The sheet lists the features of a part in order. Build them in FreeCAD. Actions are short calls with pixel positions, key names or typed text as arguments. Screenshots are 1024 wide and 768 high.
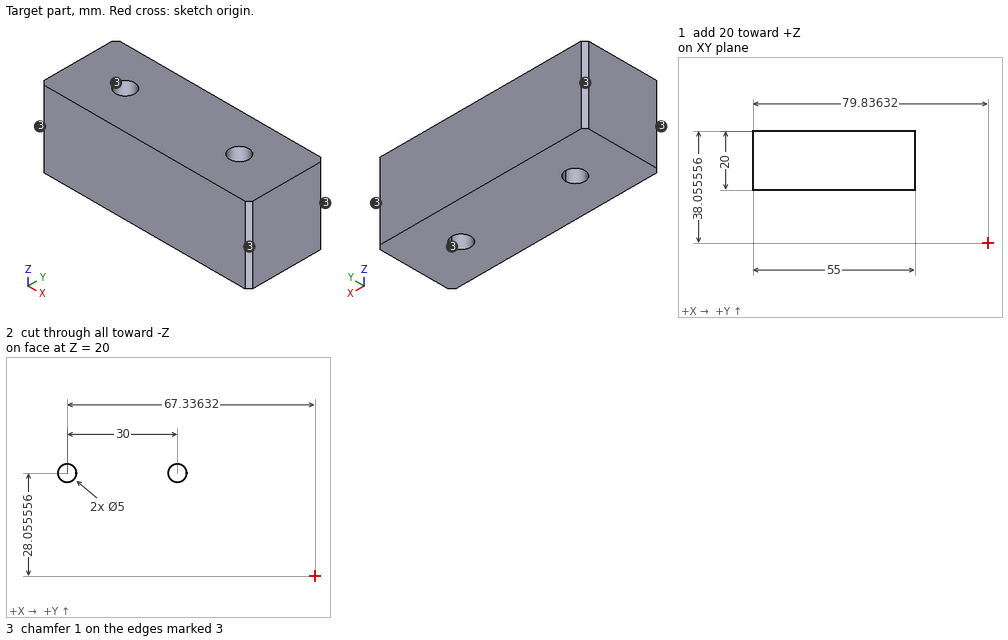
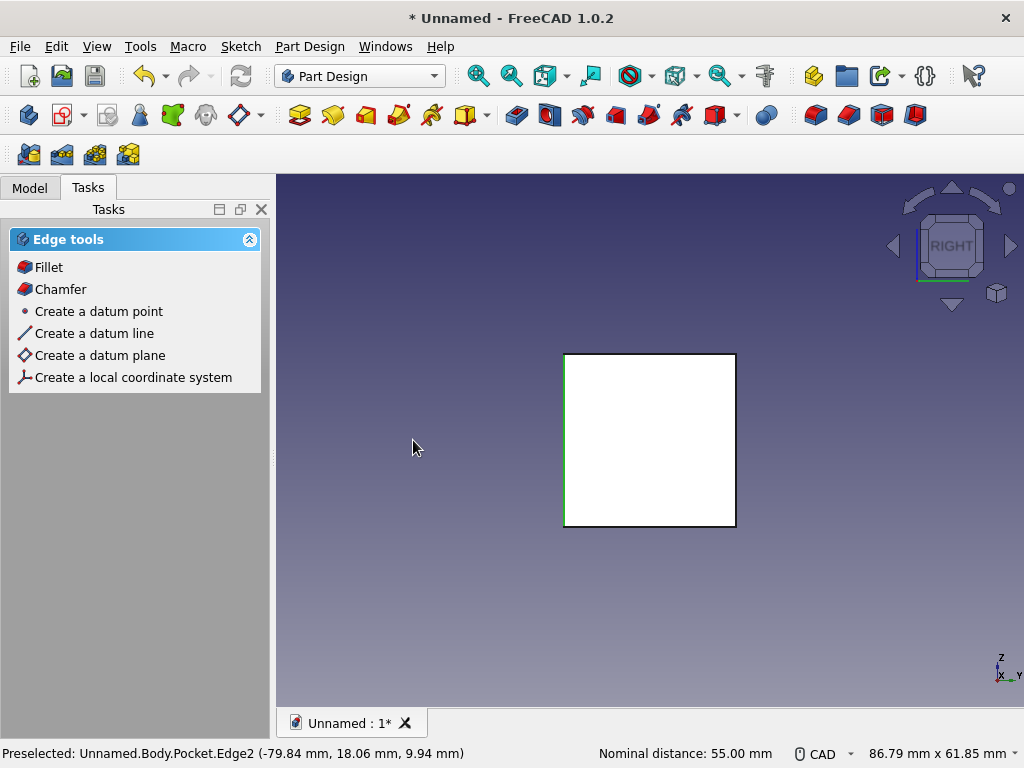
click(479, 76)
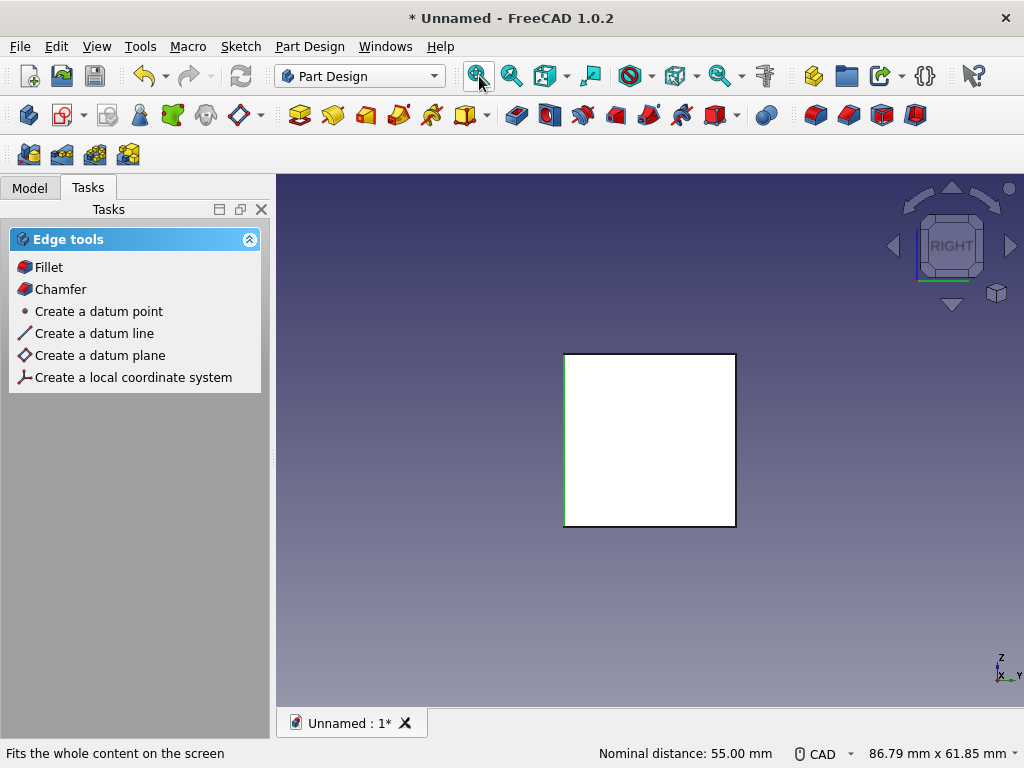
click(736, 439, ctrl)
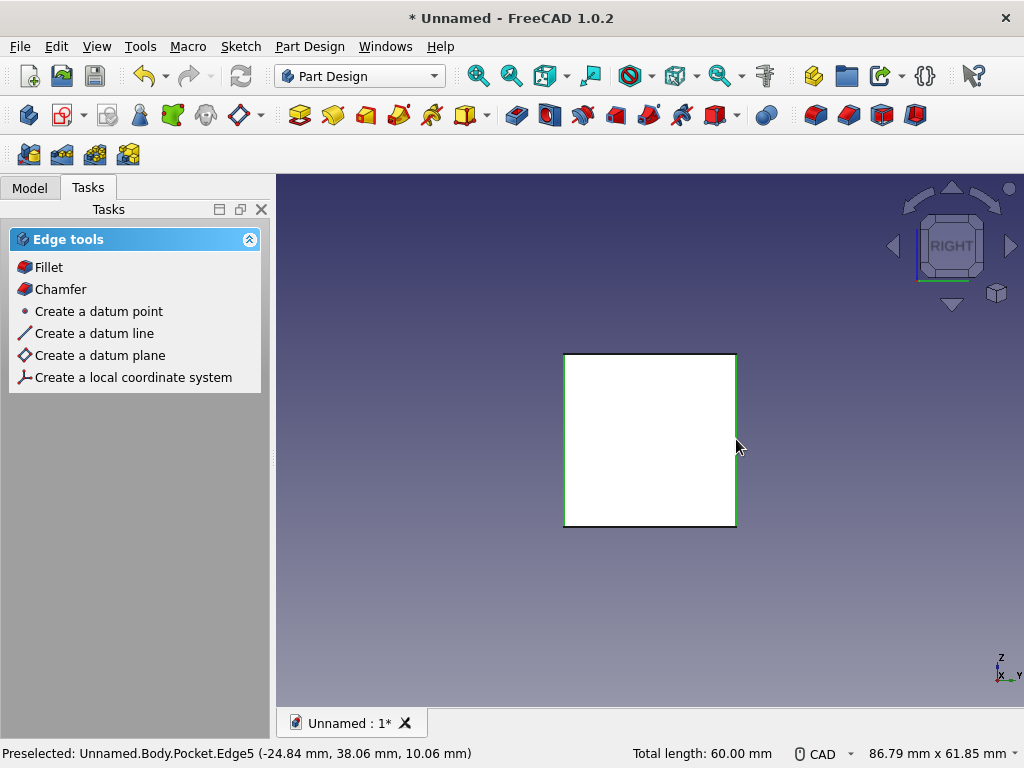
key(5)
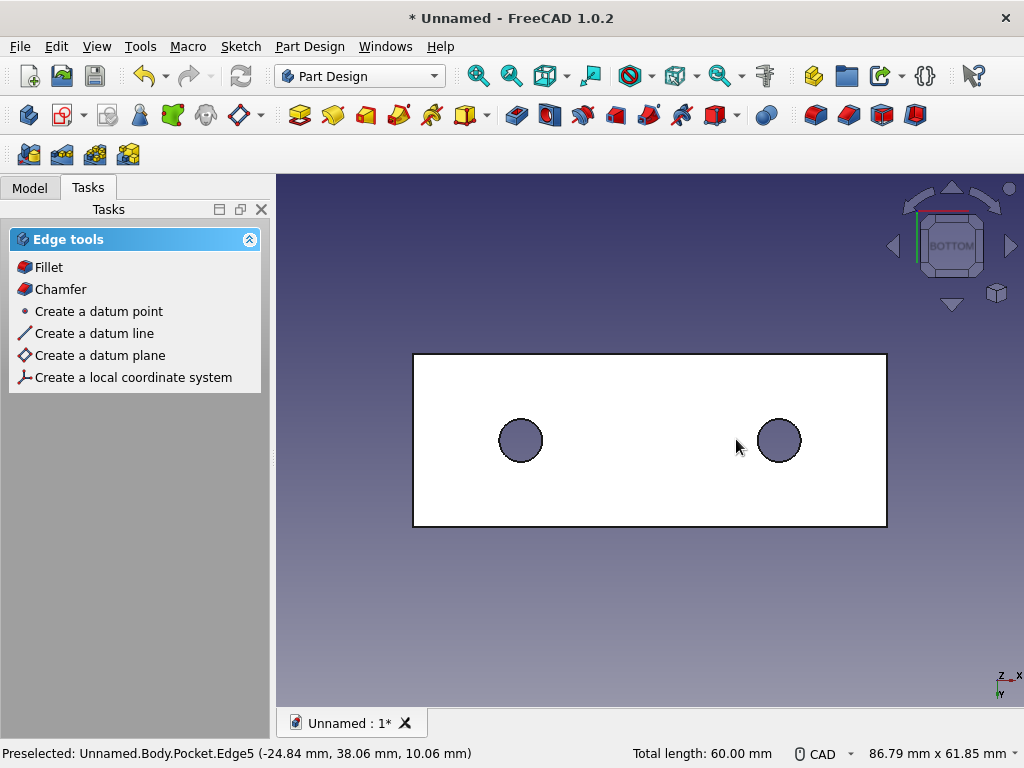
key(4)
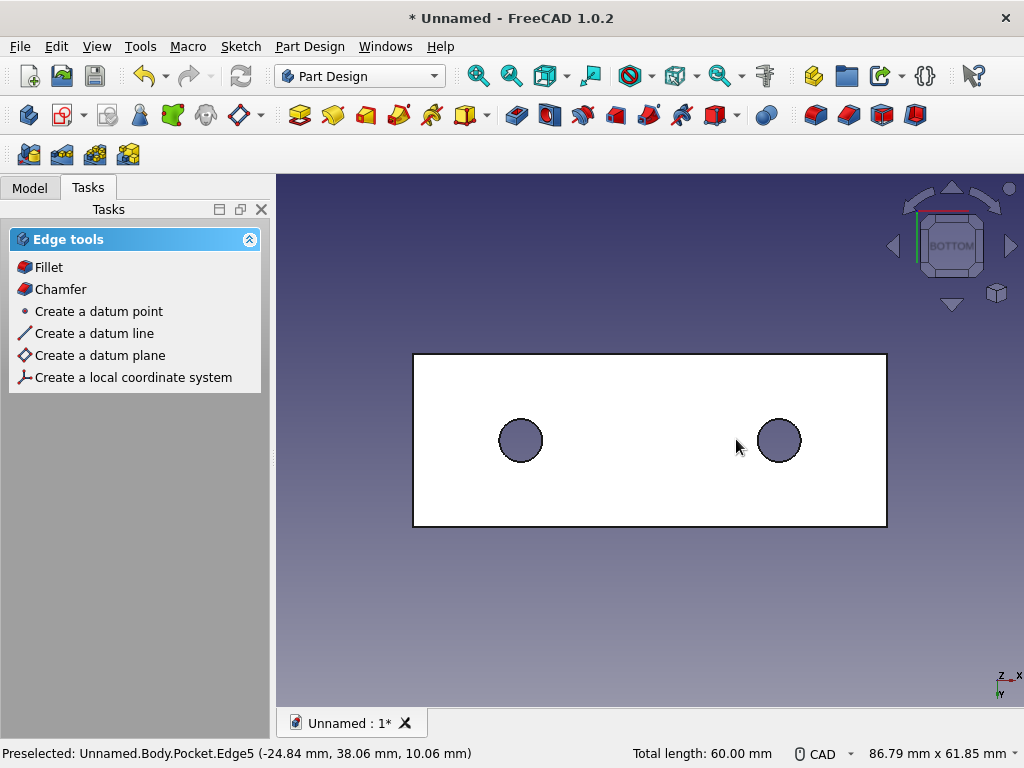
click(887, 439, ctrl)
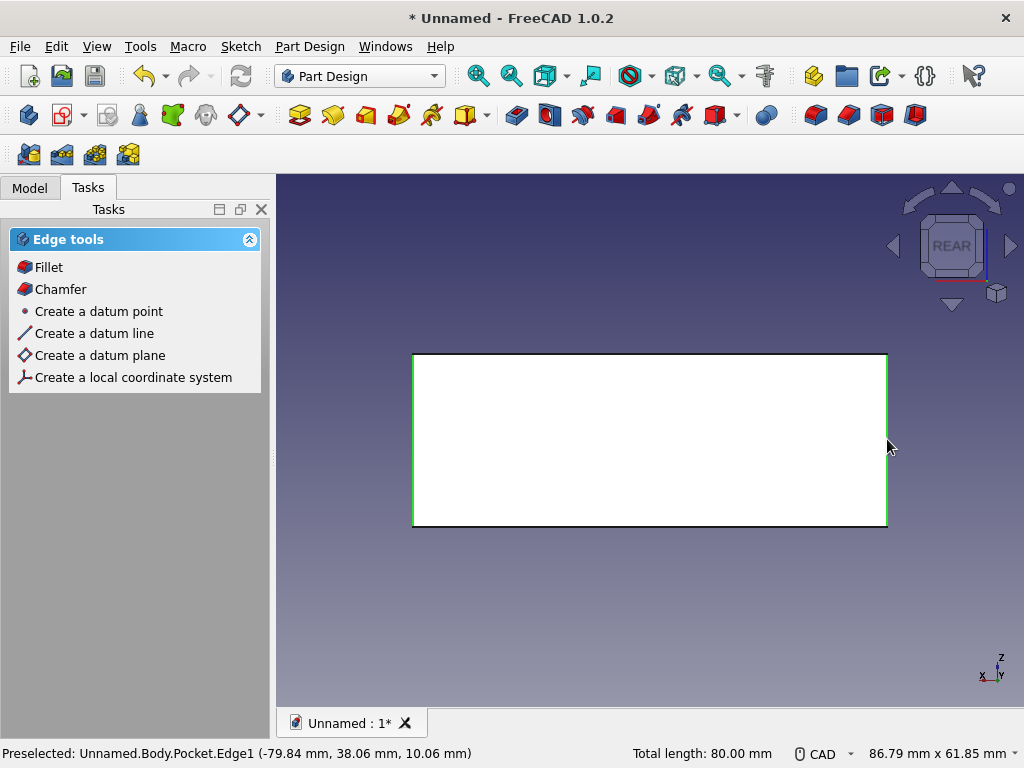
click(849, 116)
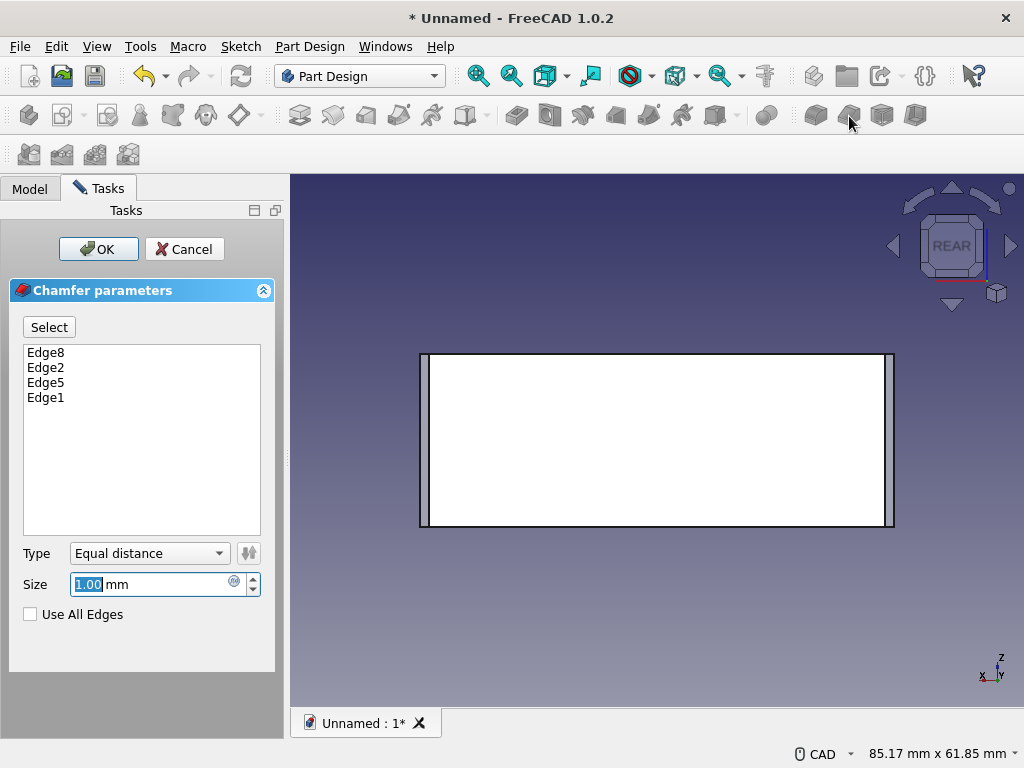
text(1)
key(Tab)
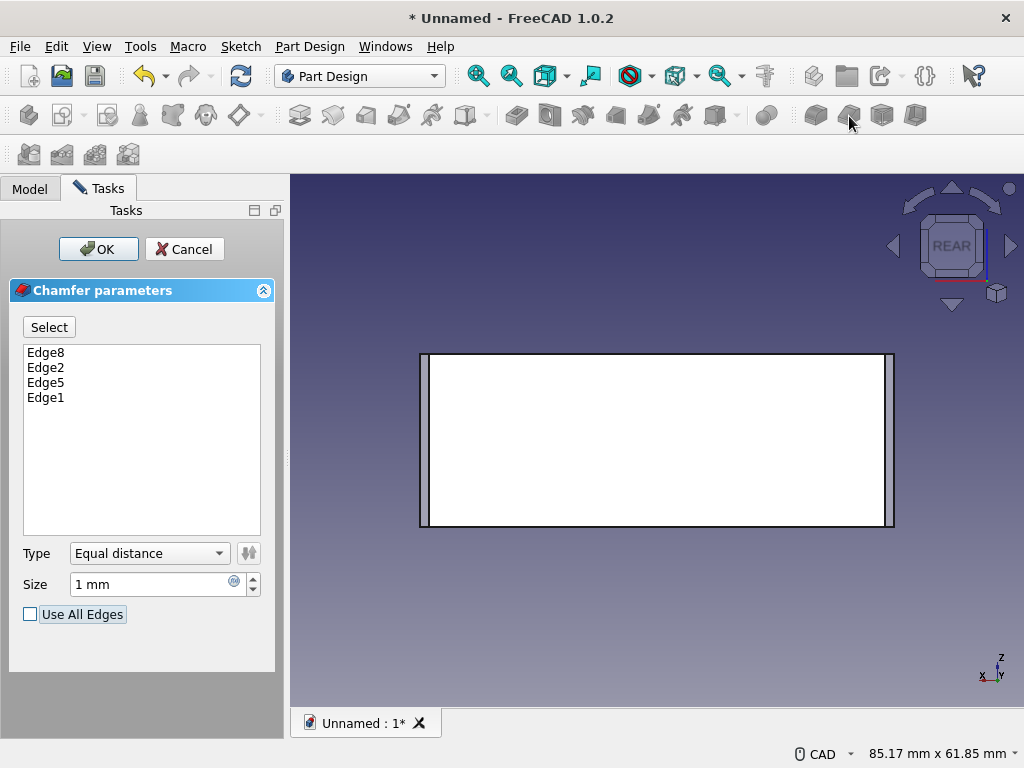
click(99, 249)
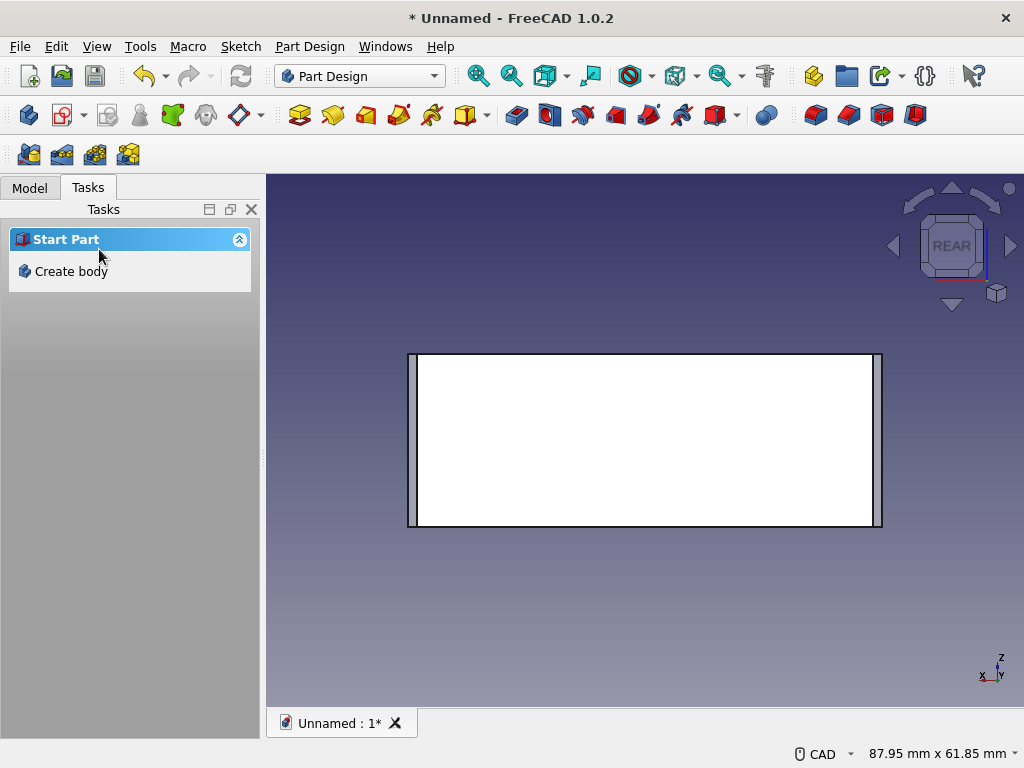
key(0)